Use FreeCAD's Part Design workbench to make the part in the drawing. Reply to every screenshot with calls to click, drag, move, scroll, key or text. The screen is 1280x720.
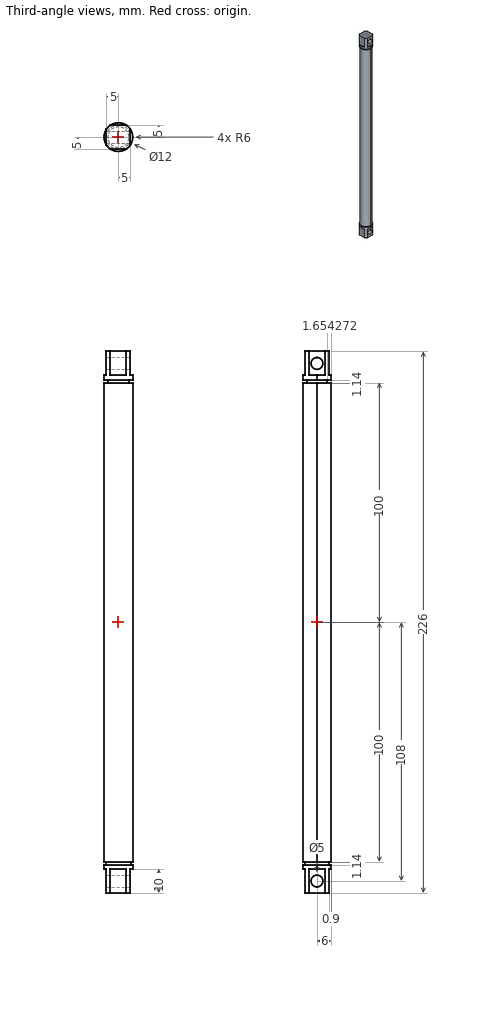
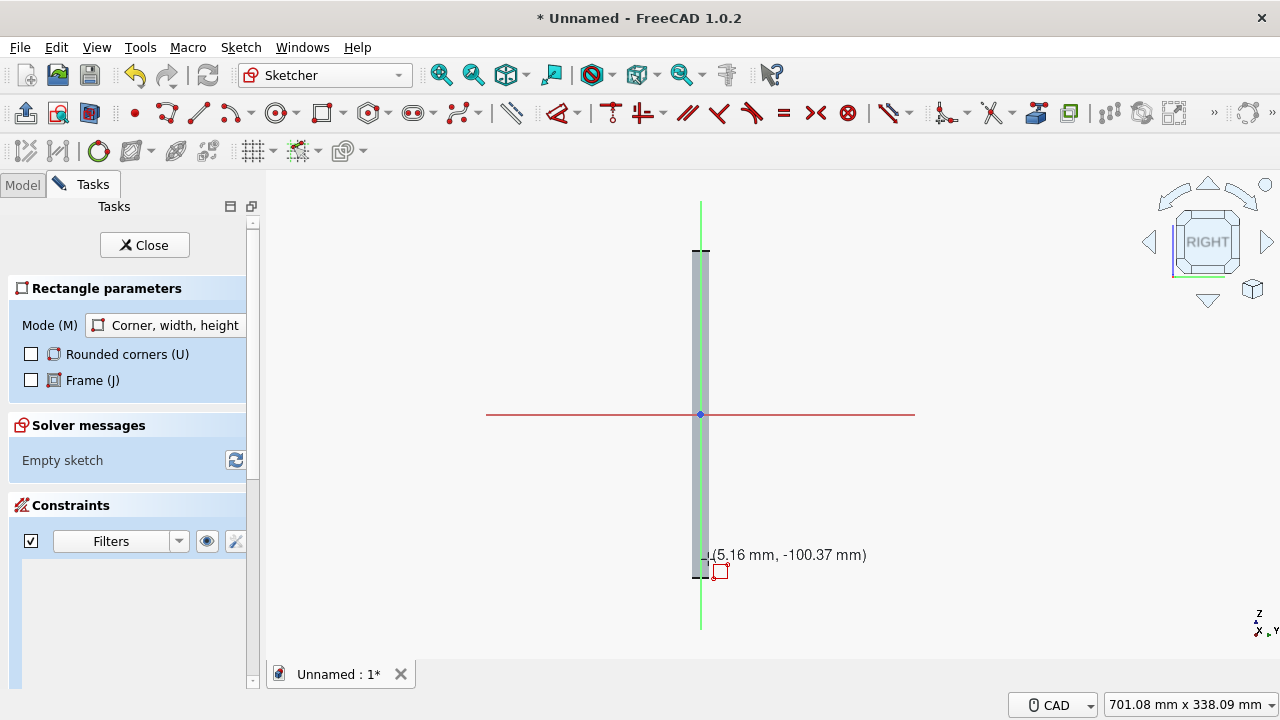
scroll(708, 559, up, 4)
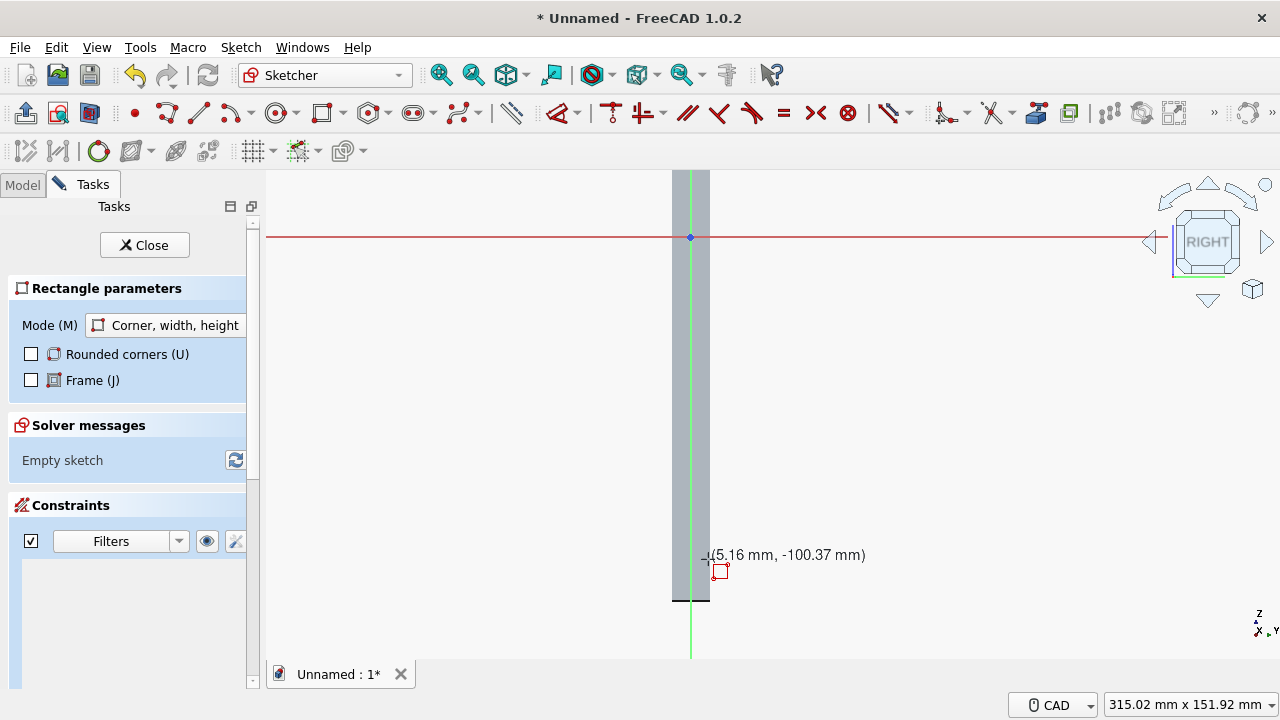
click(707, 559)
move(710, 563)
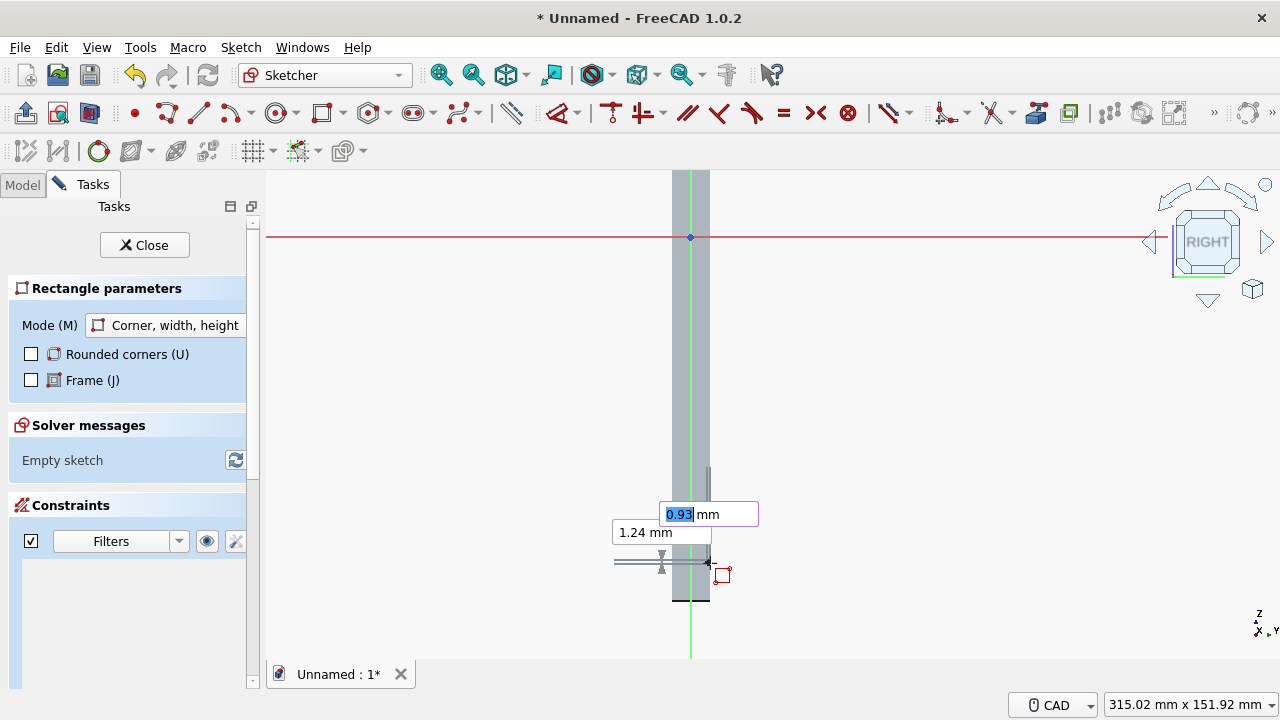
text(0.9)
key(Tab)
text(1.14)
key(Return)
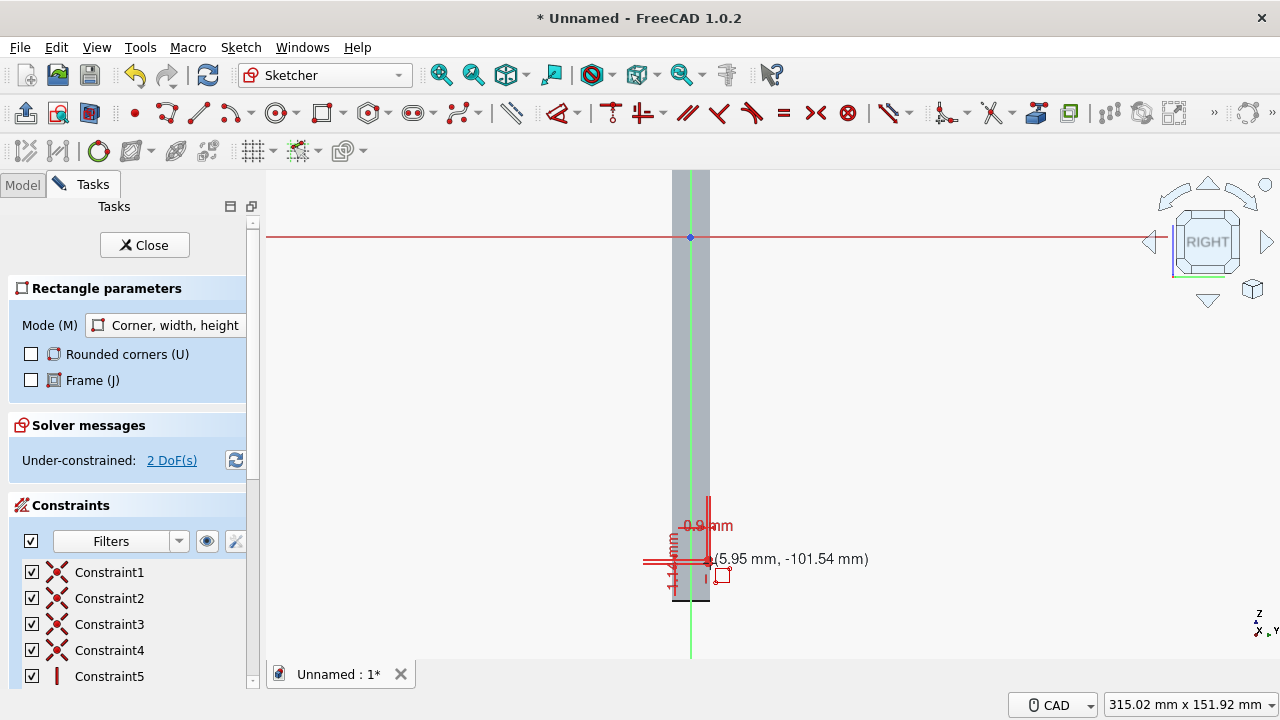
scroll(708, 559, down, 4)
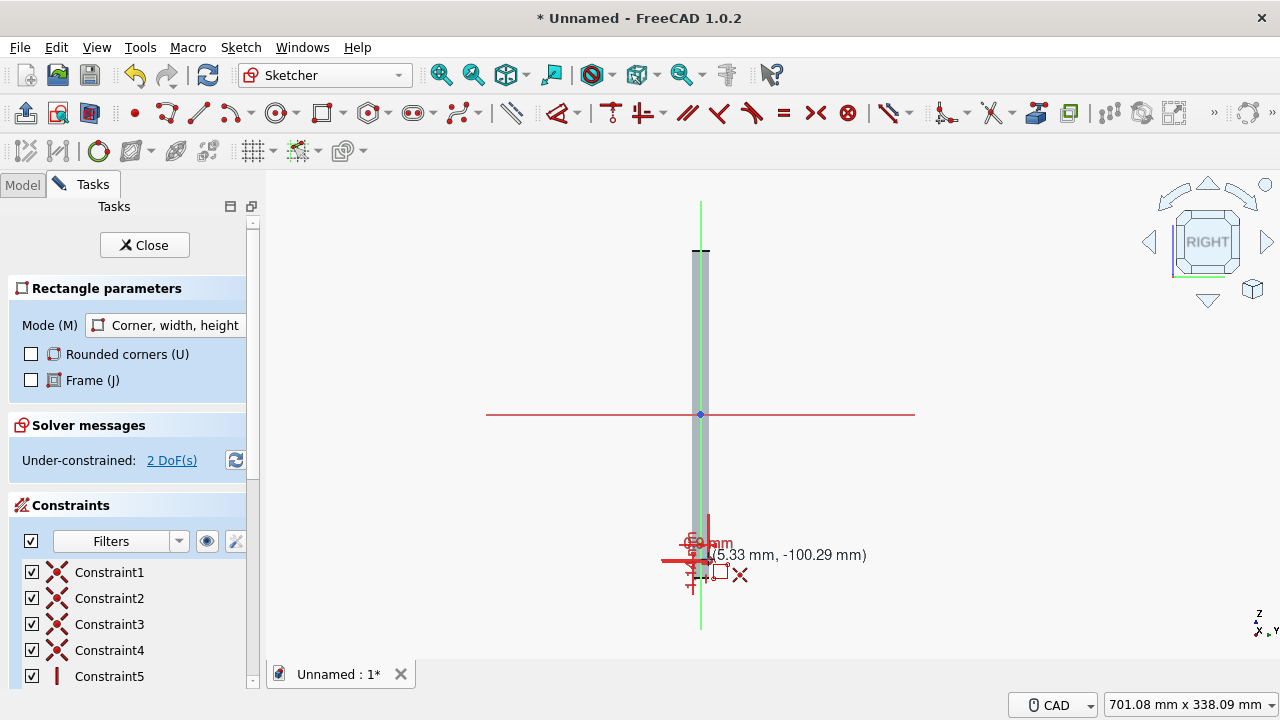
scroll(707, 269, up, 12)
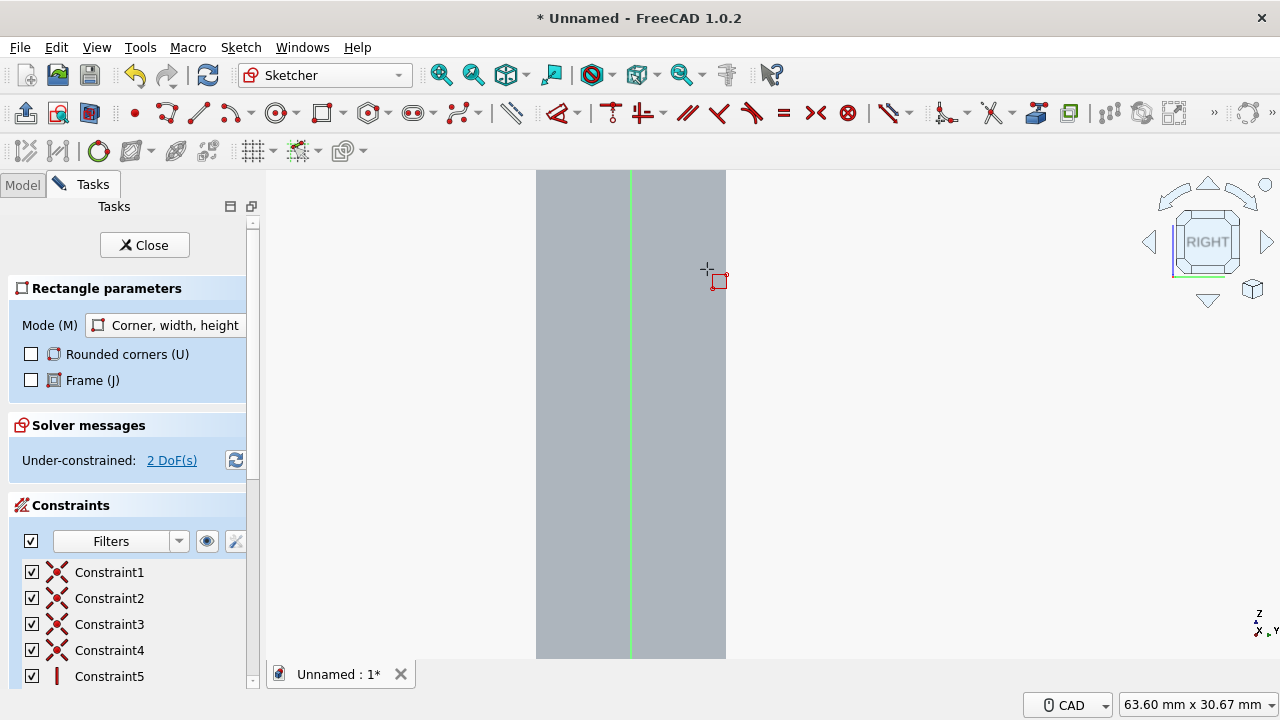
scroll(707, 269, down, 12)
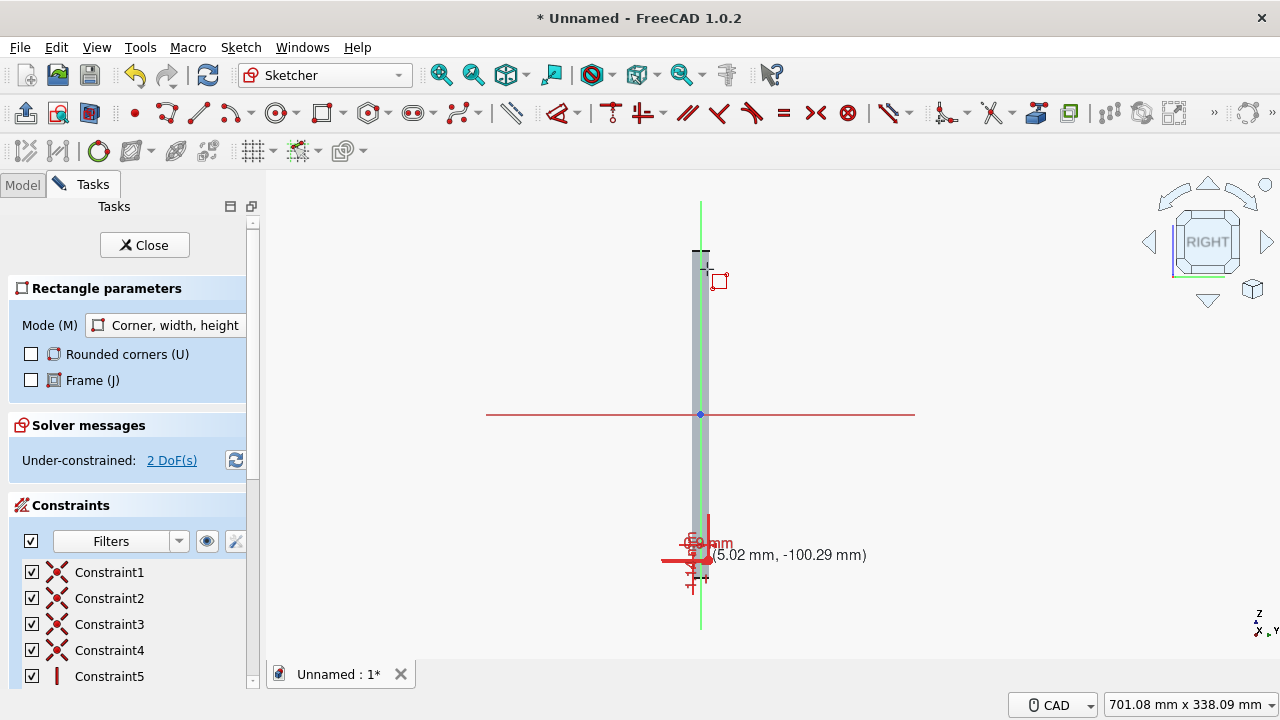
scroll(707, 269, up, 5)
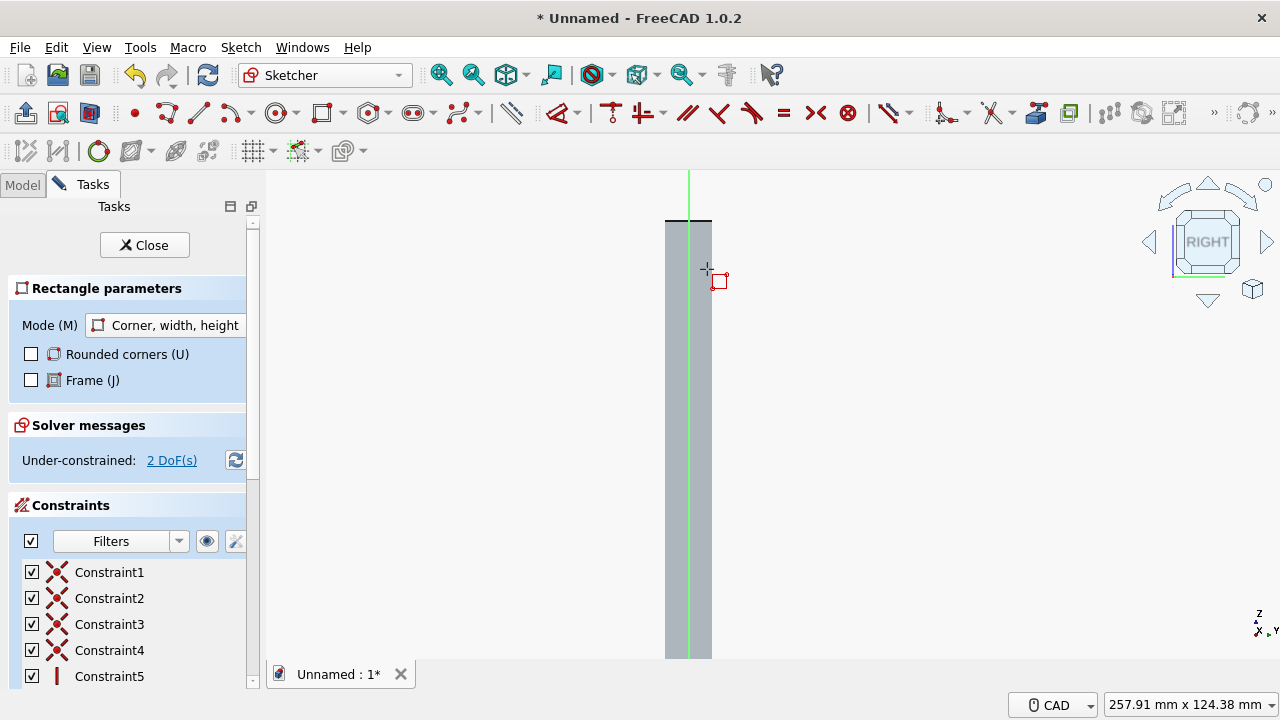
click(706, 267)
move(712, 272)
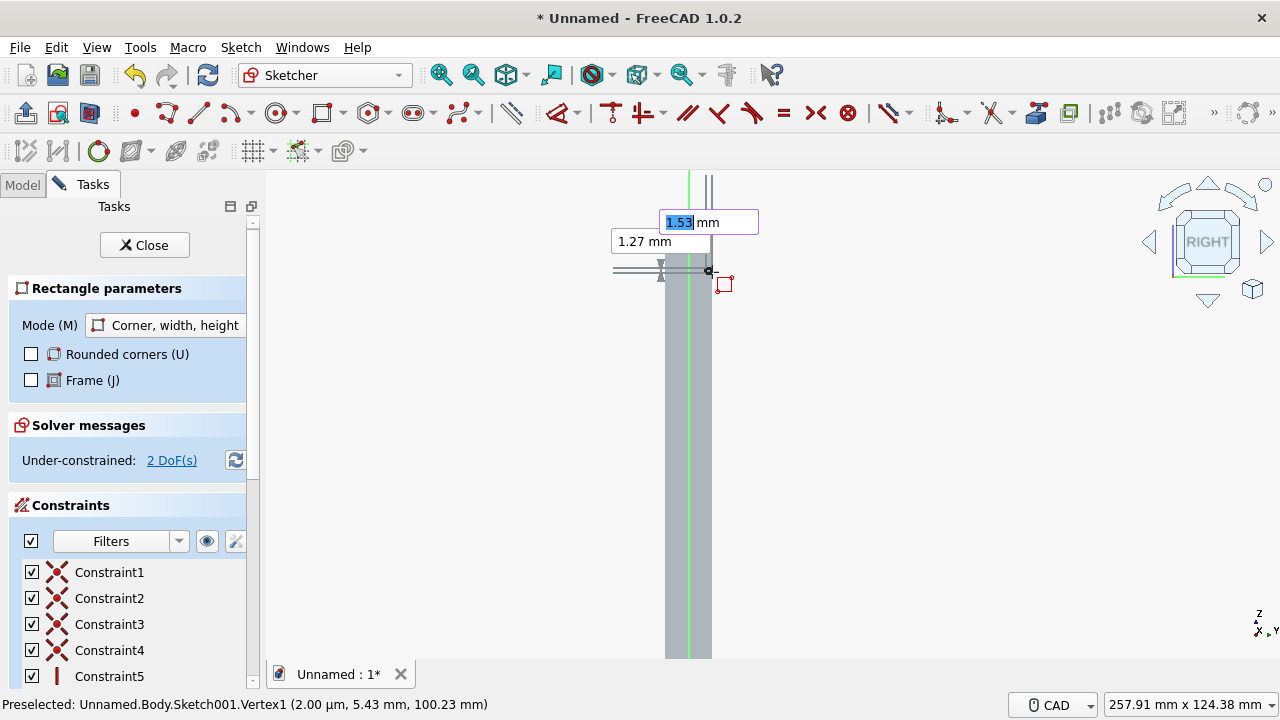
text(1.654272)
key(Tab)
text(1.14)
key(Return)
key(Escape)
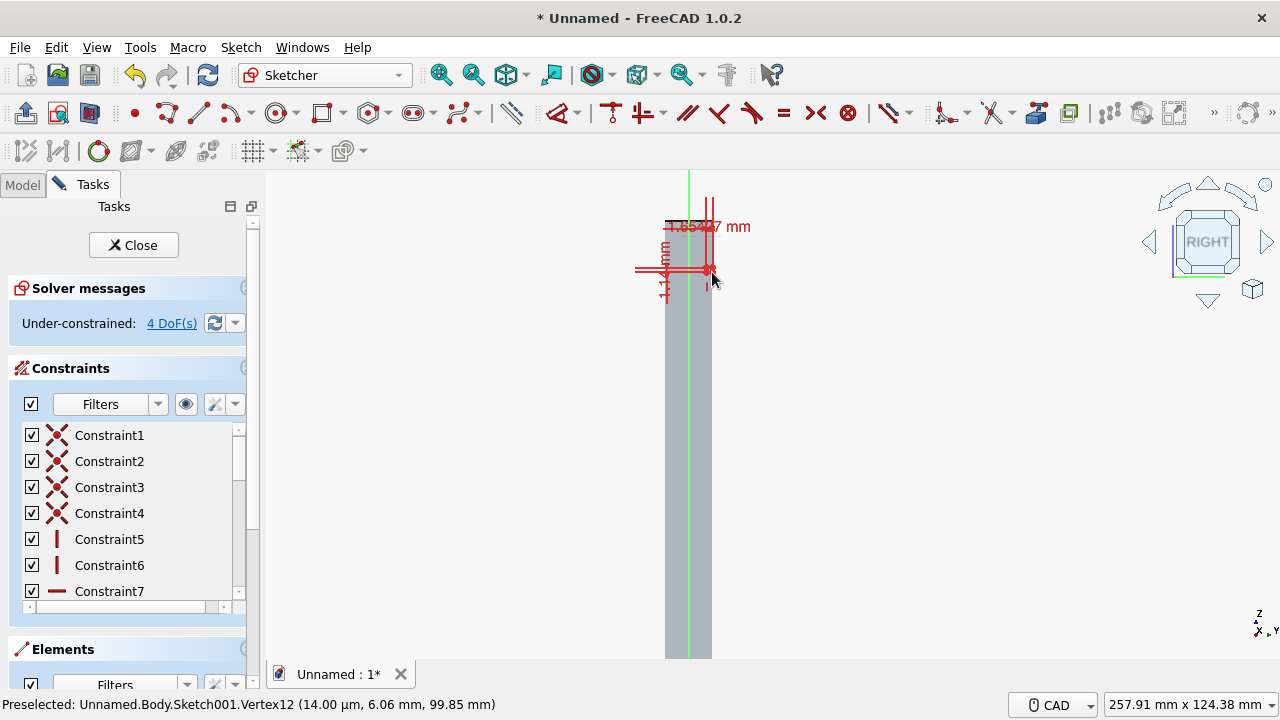
key(d)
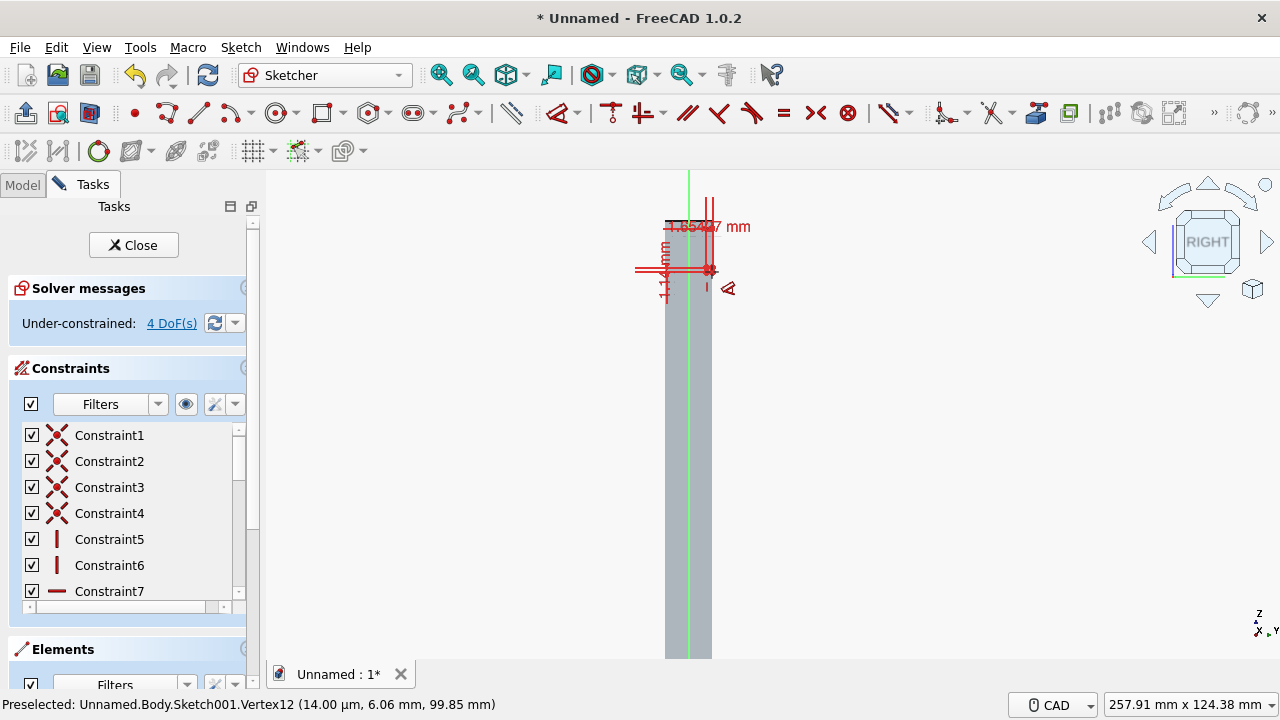
scroll(707, 269, down, 5)